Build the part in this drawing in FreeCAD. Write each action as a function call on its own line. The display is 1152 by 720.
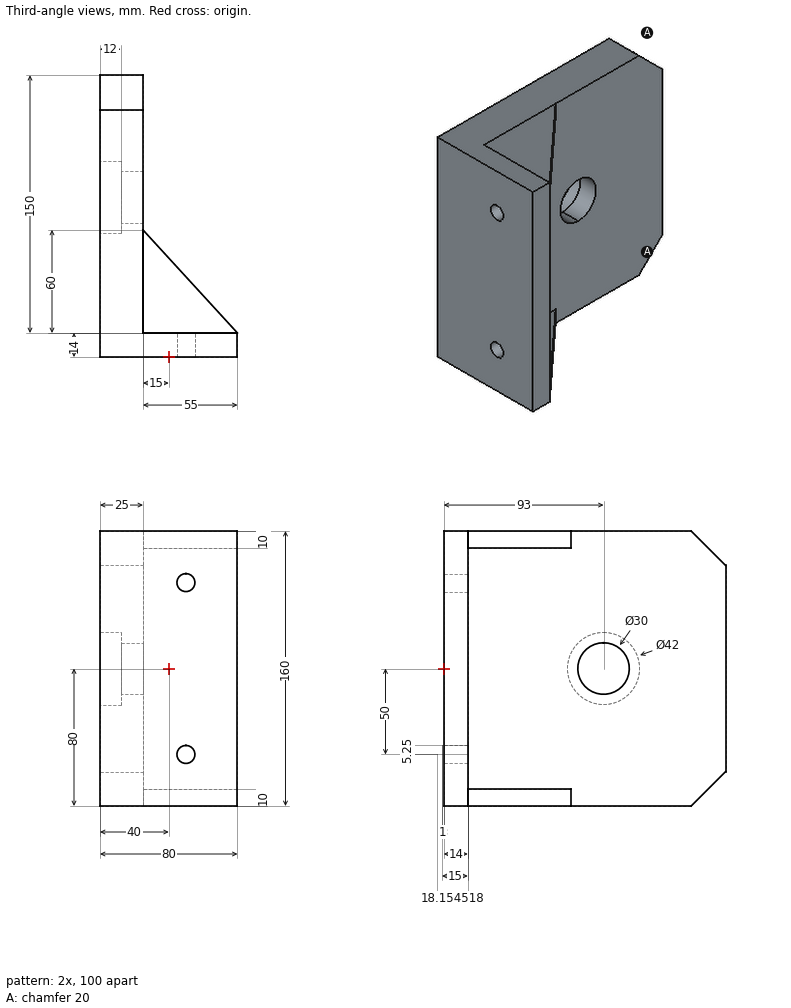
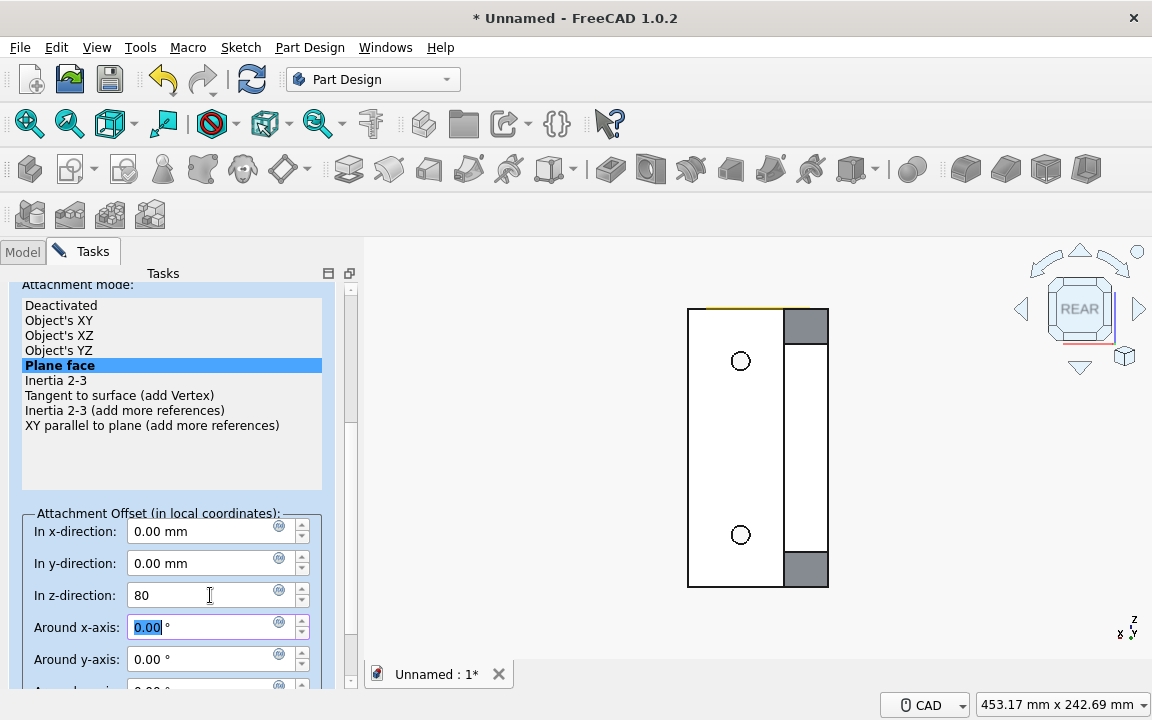
scroll(351, 486, up, 5)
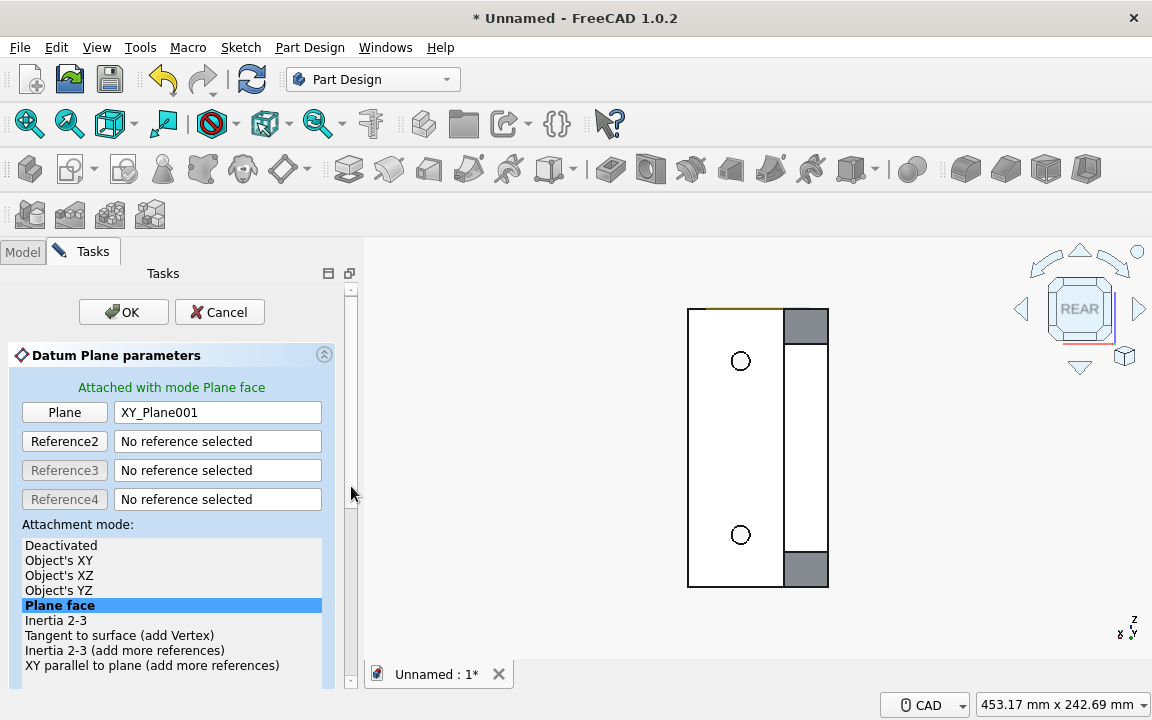
click(124, 312)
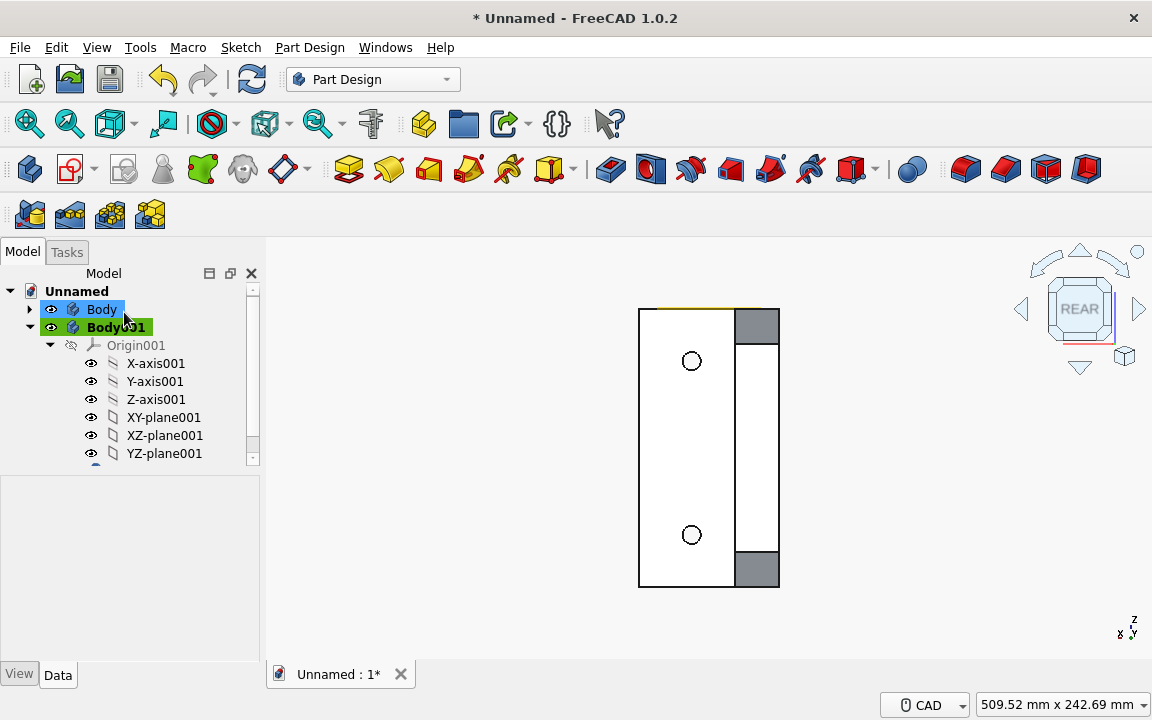
scroll(100, 377, down, 3)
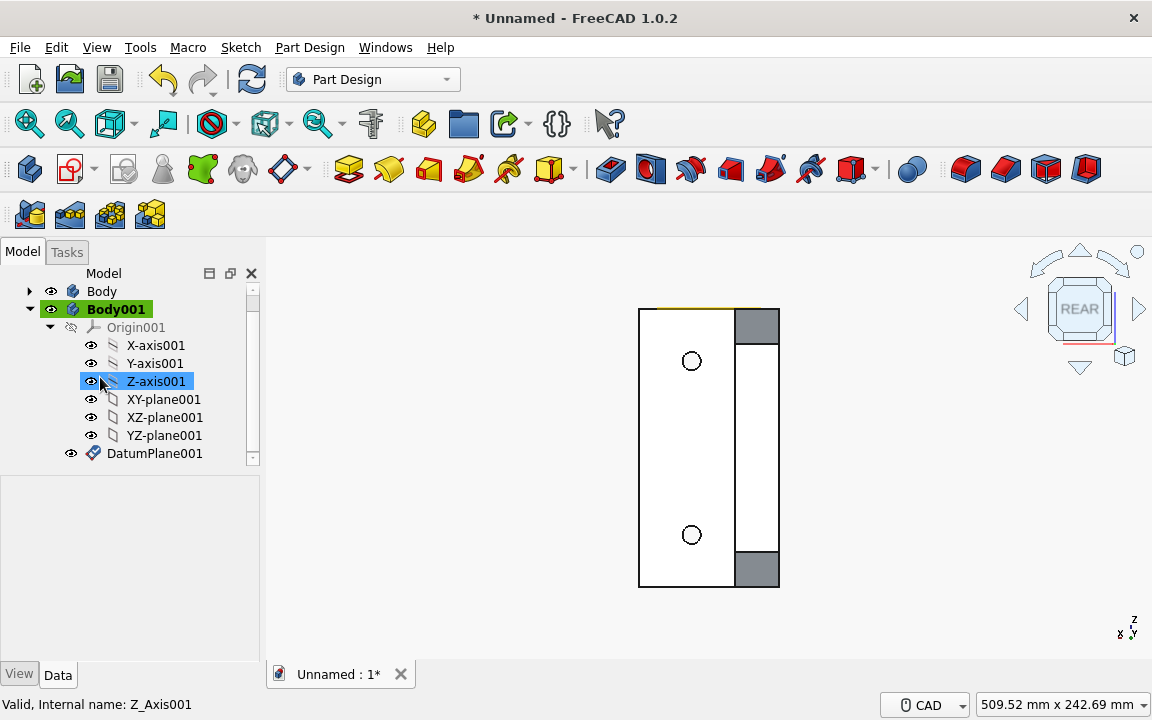
click(116, 453)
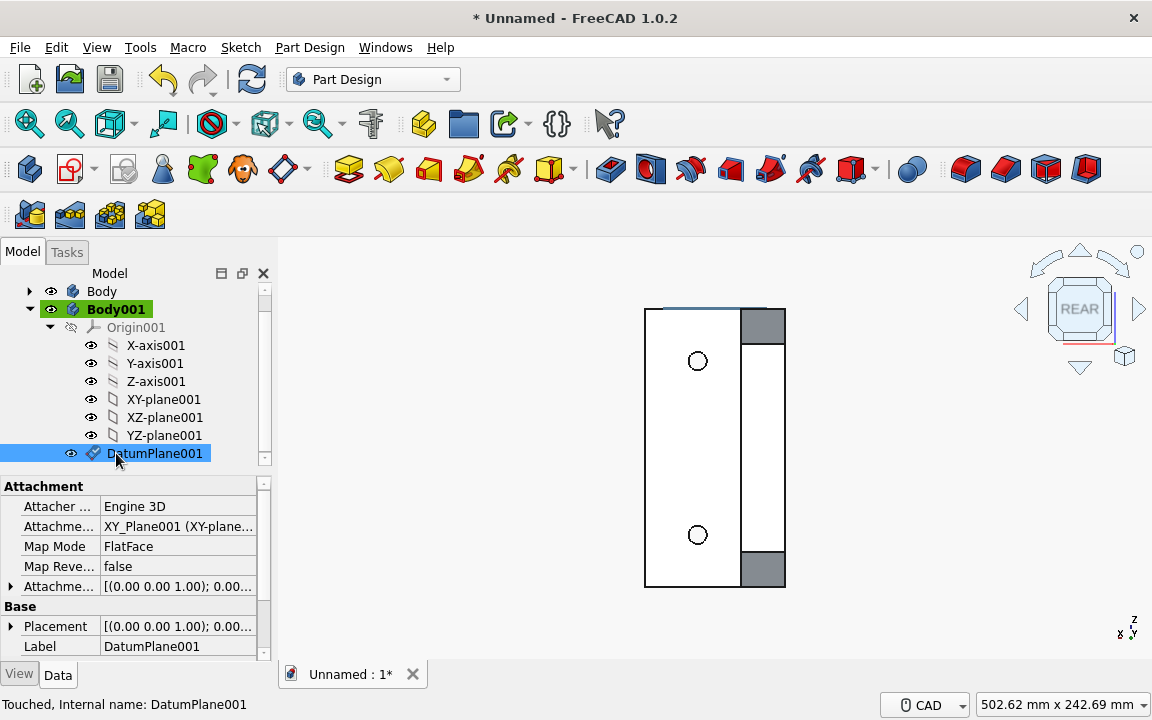
click(70, 170)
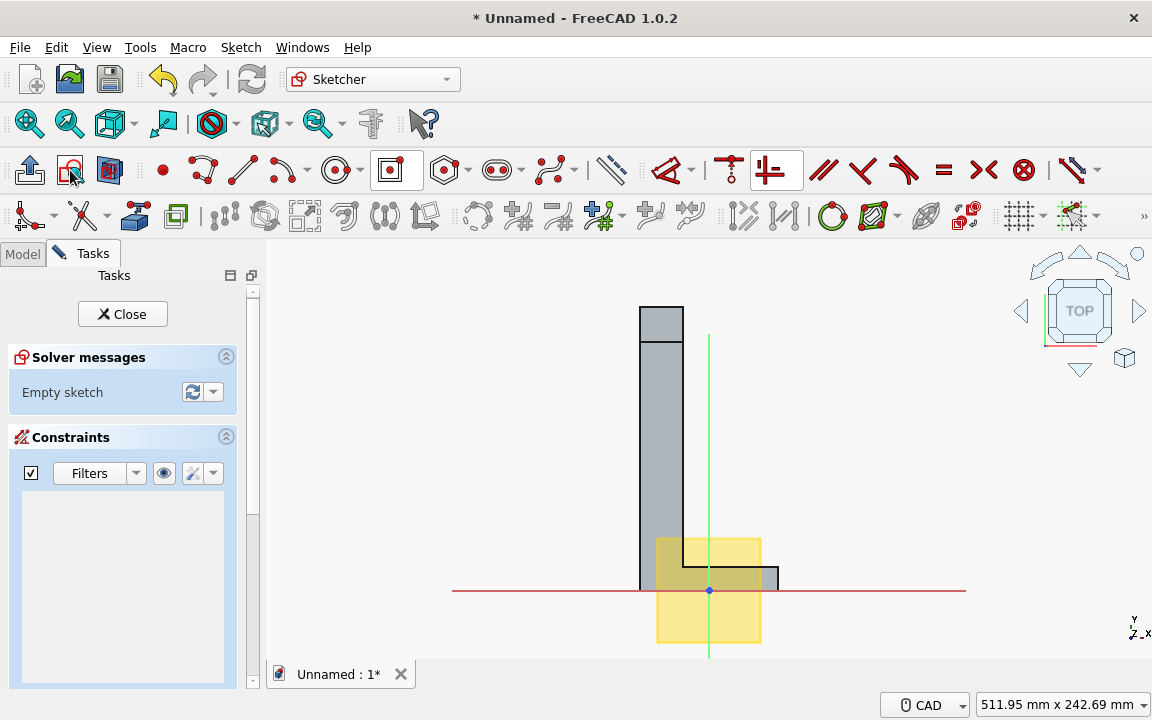
scroll(840, 622, up, 3)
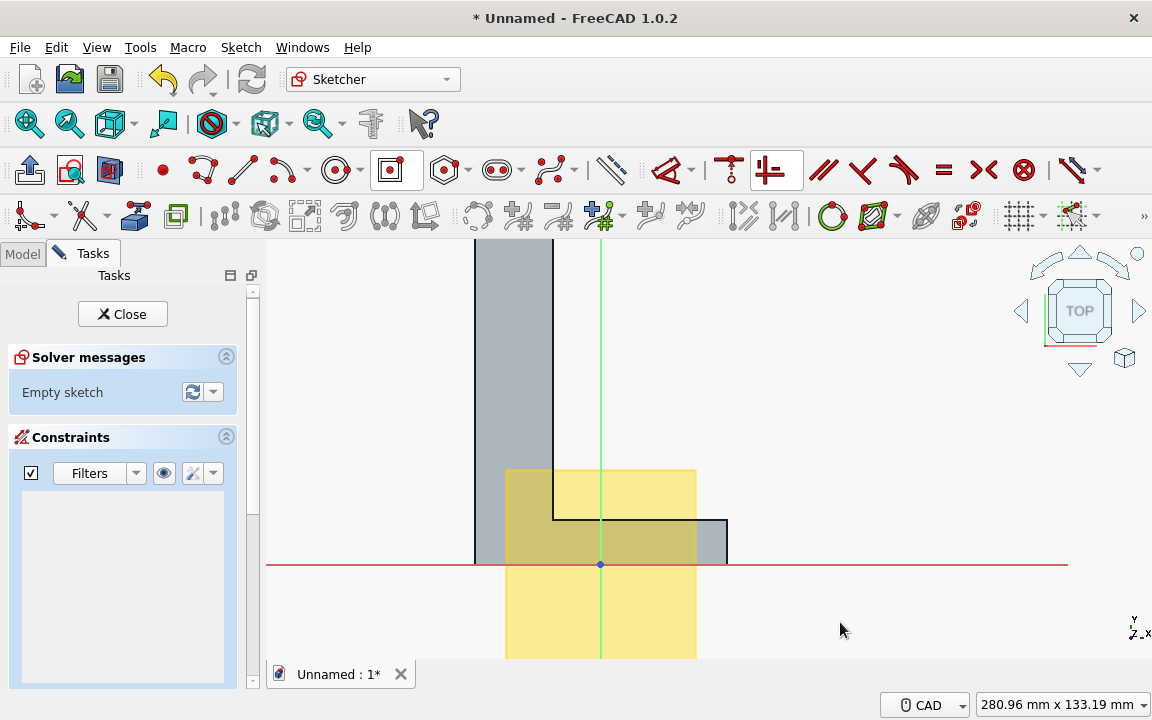
click(204, 170)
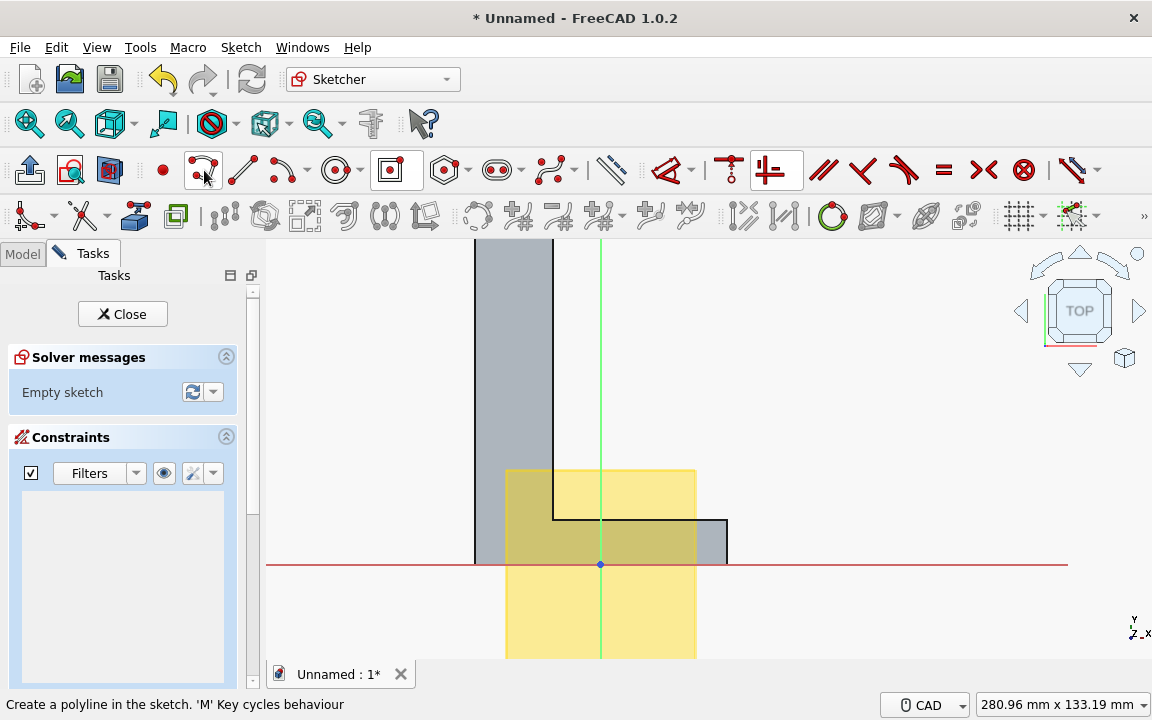
click(553, 520)
click(727, 520)
click(553, 331)
click(553, 521)
key(Escape)
key(Escape)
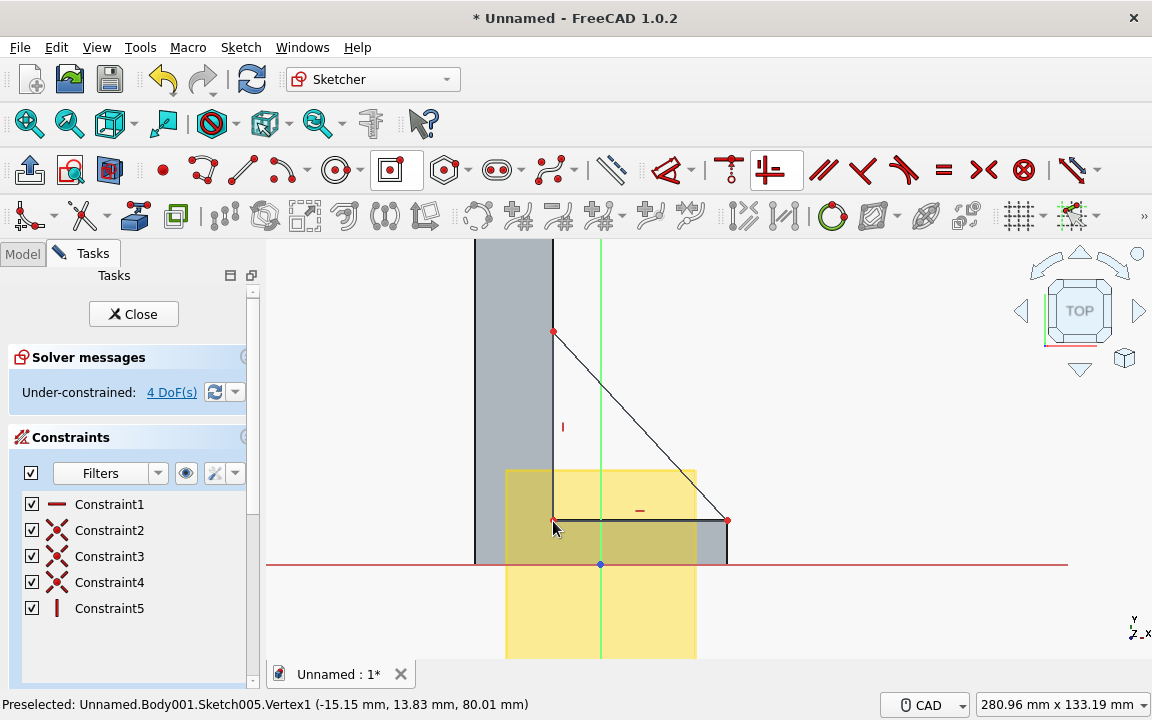
click(666, 170)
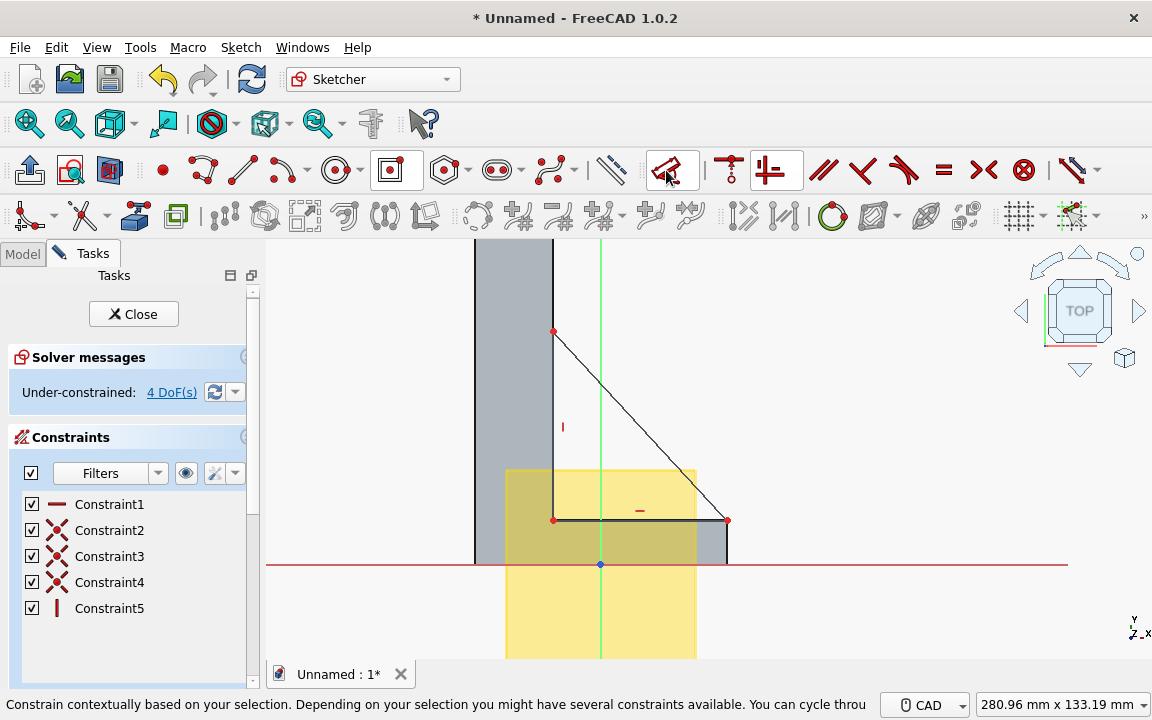
click(675, 521)
click(640, 487)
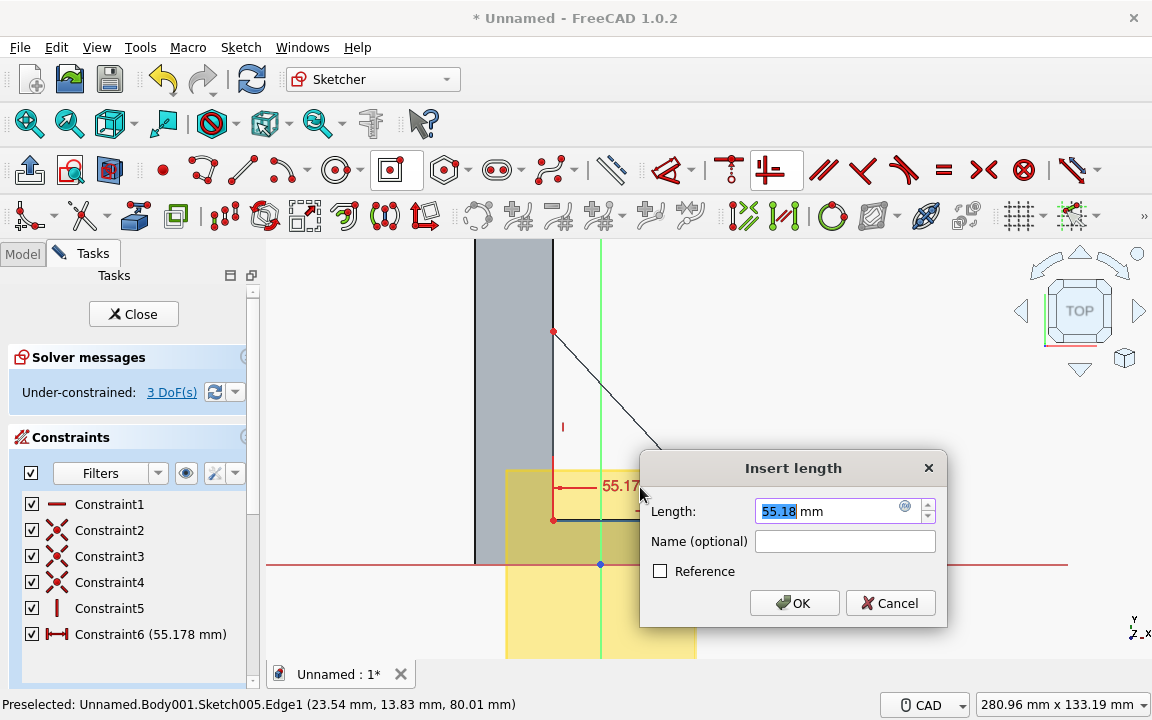
text(55)
key(Return)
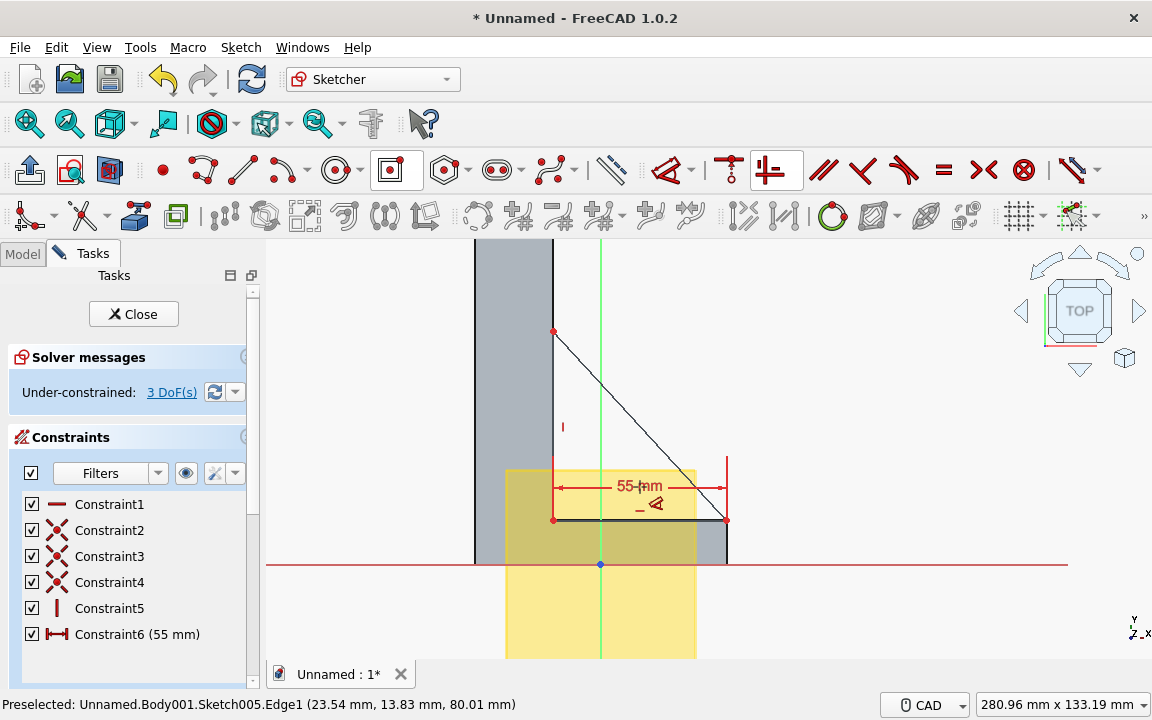
click(553, 389)
click(519, 427)